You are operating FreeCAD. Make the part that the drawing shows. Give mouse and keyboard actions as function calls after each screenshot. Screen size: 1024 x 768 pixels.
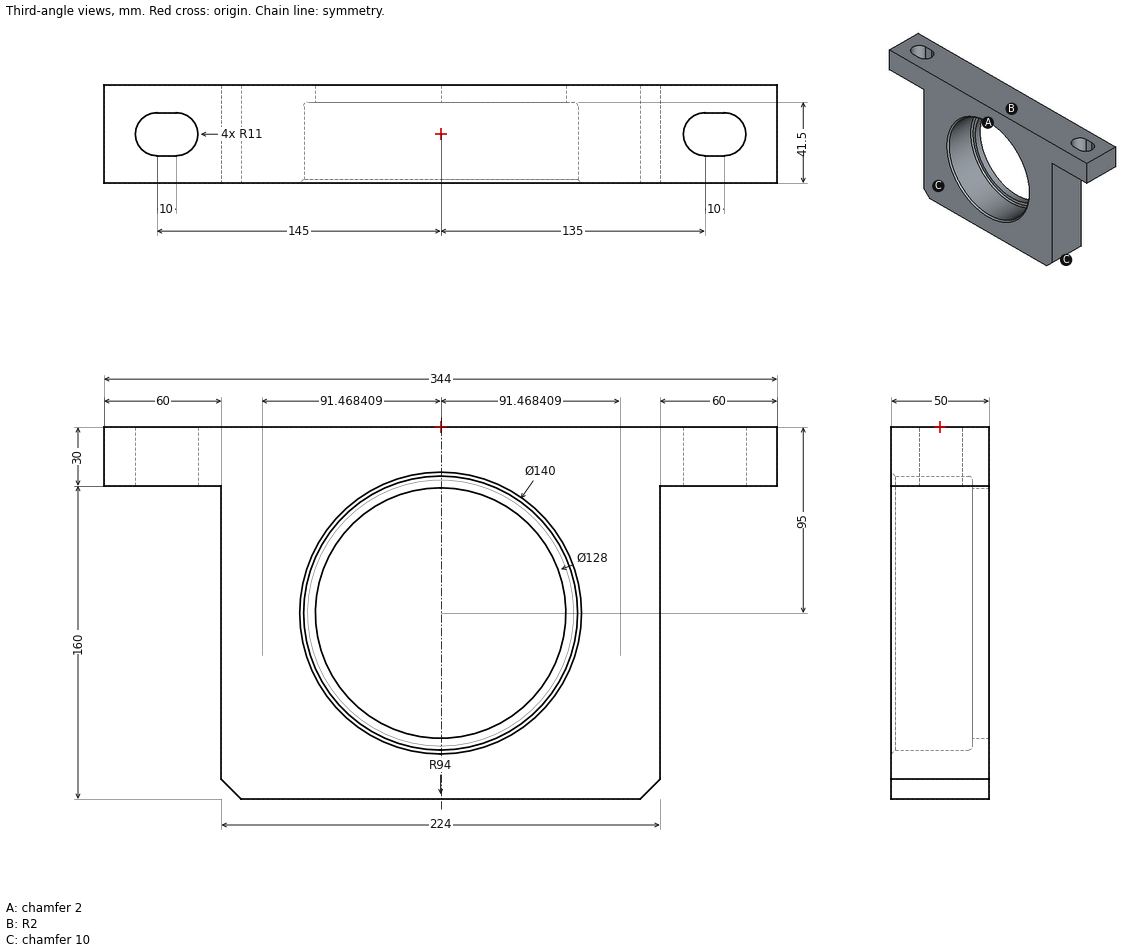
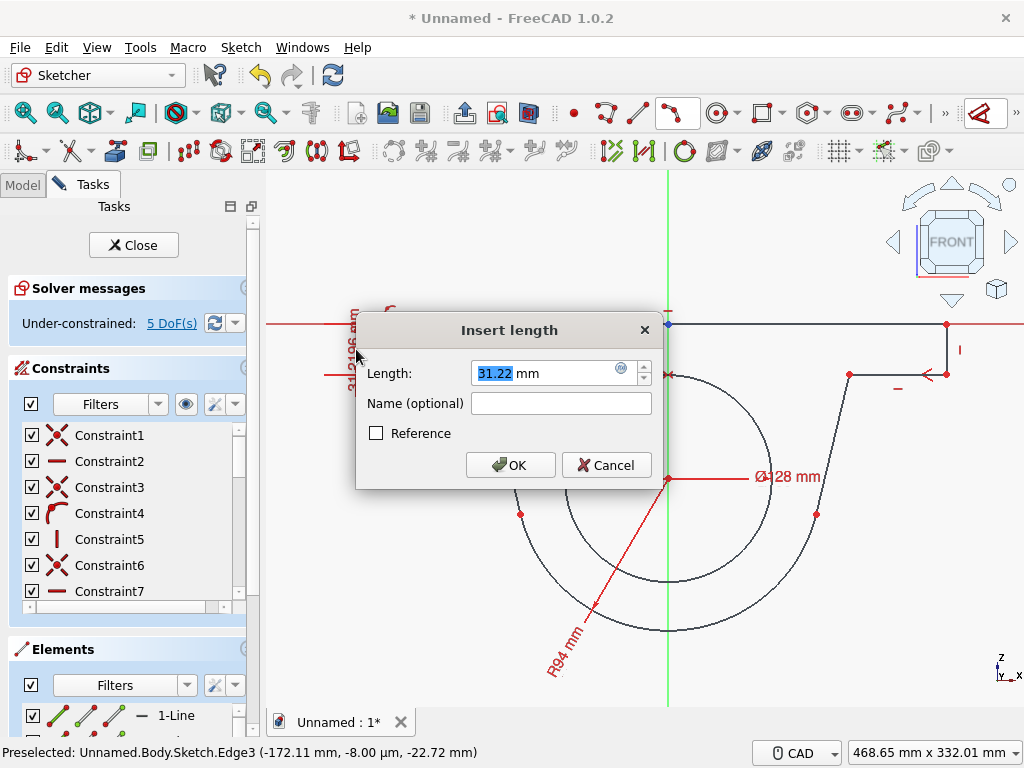
text(30)
key(Return)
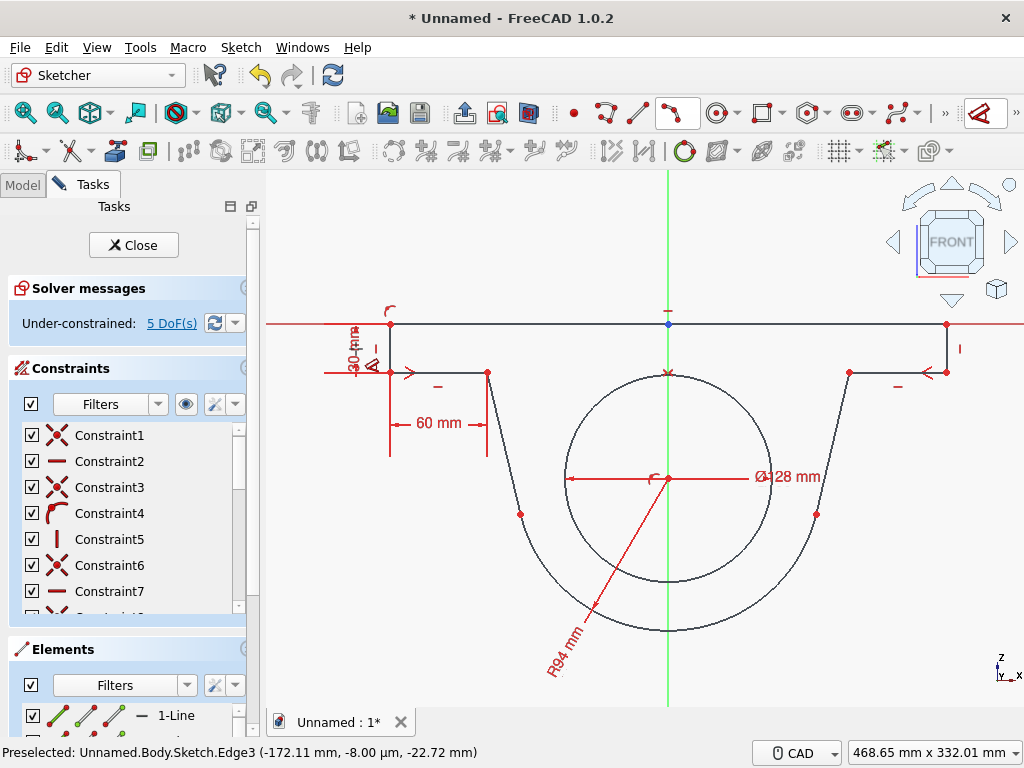
scroll(390, 360, down, 2)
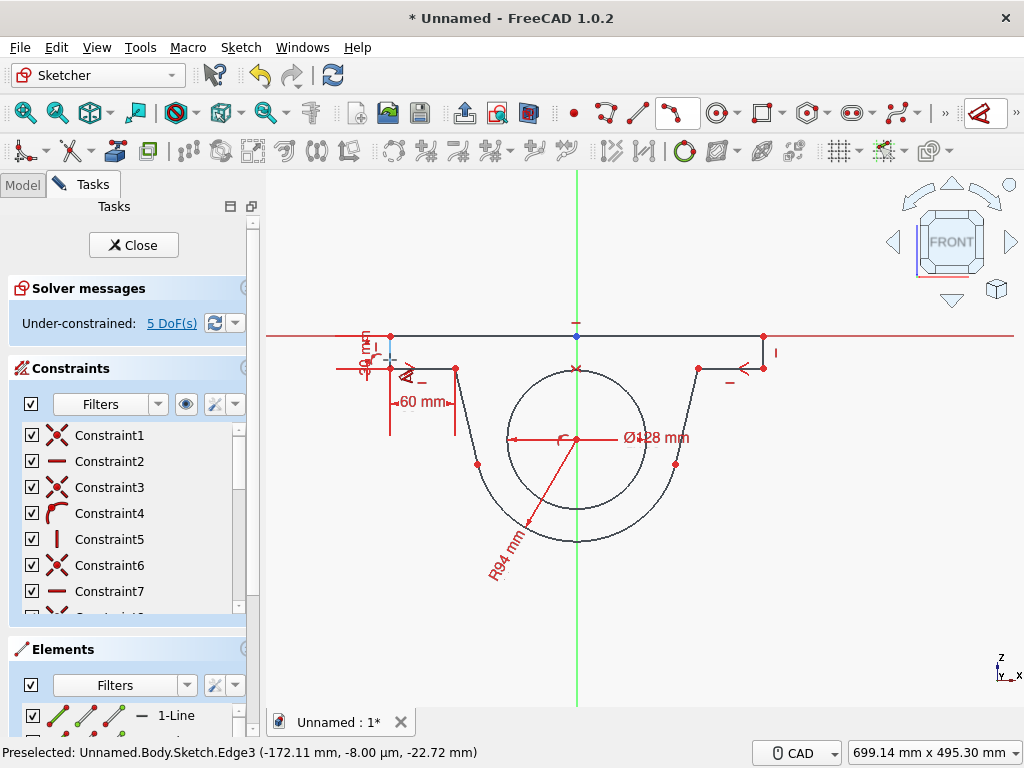
click(744, 369)
click(731, 403)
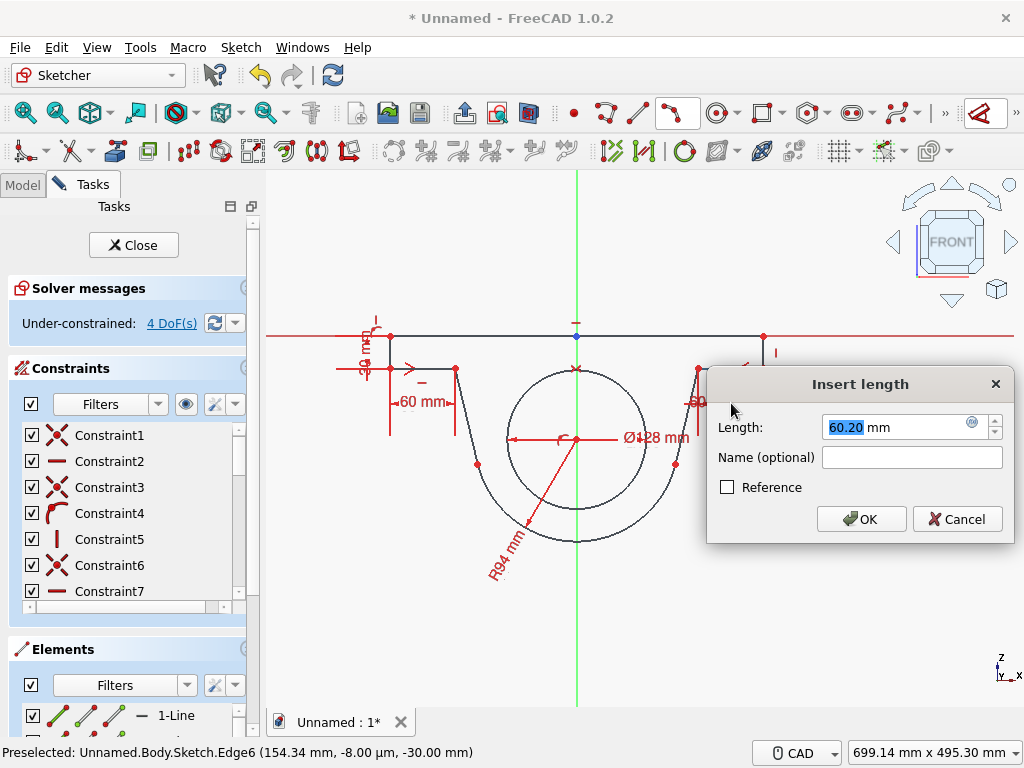
text(60)
key(Return)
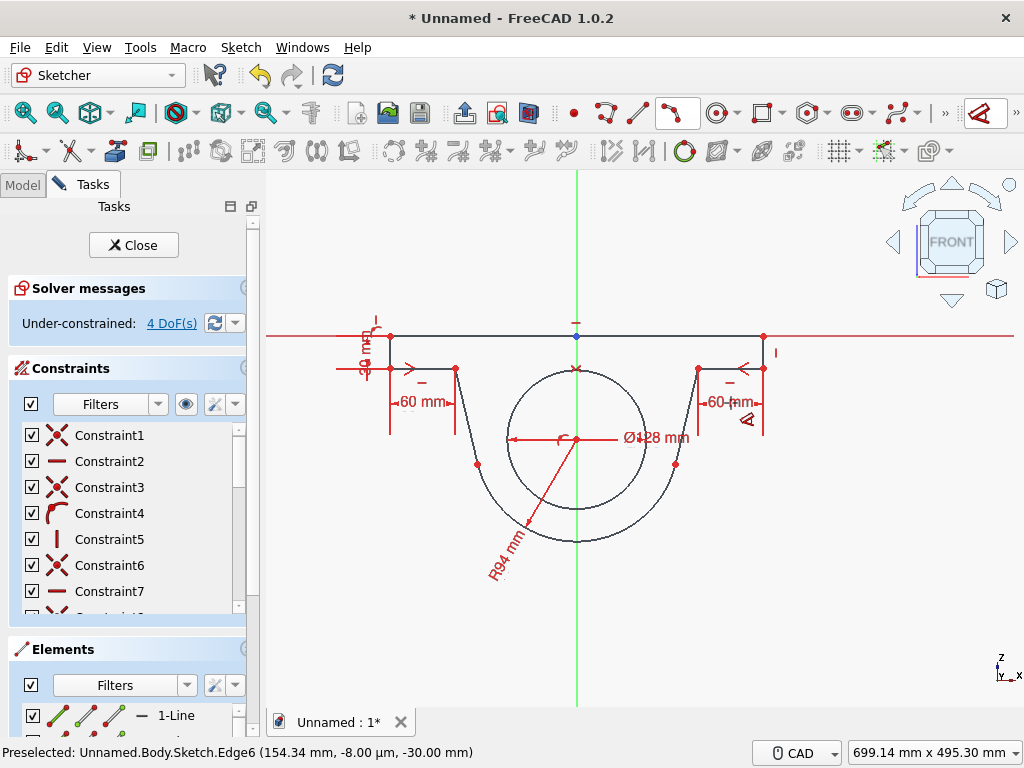
click(577, 440)
click(611, 364)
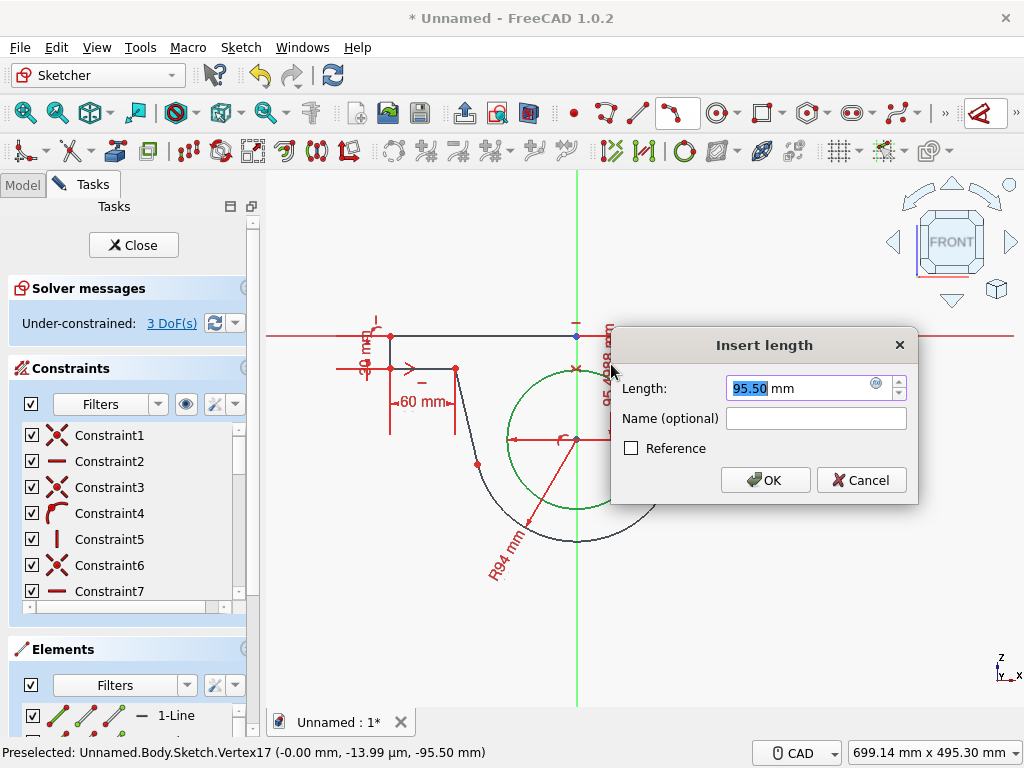
text(95)
key(Return)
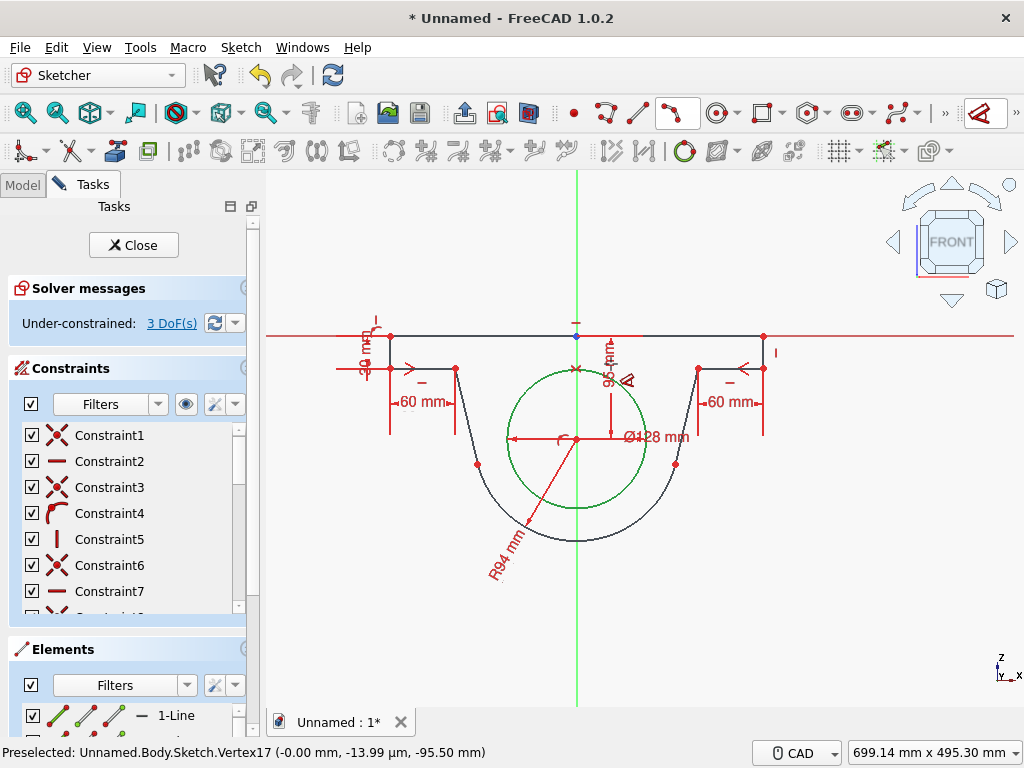
click(502, 336)
click(491, 302)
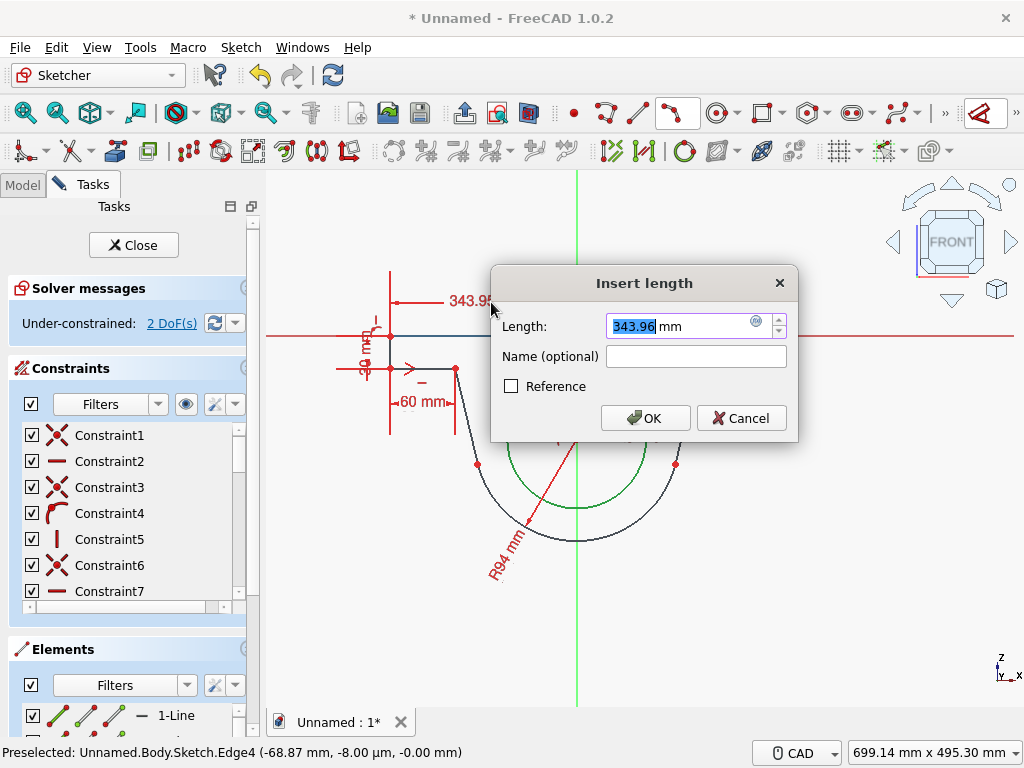
text(344)
key(Return)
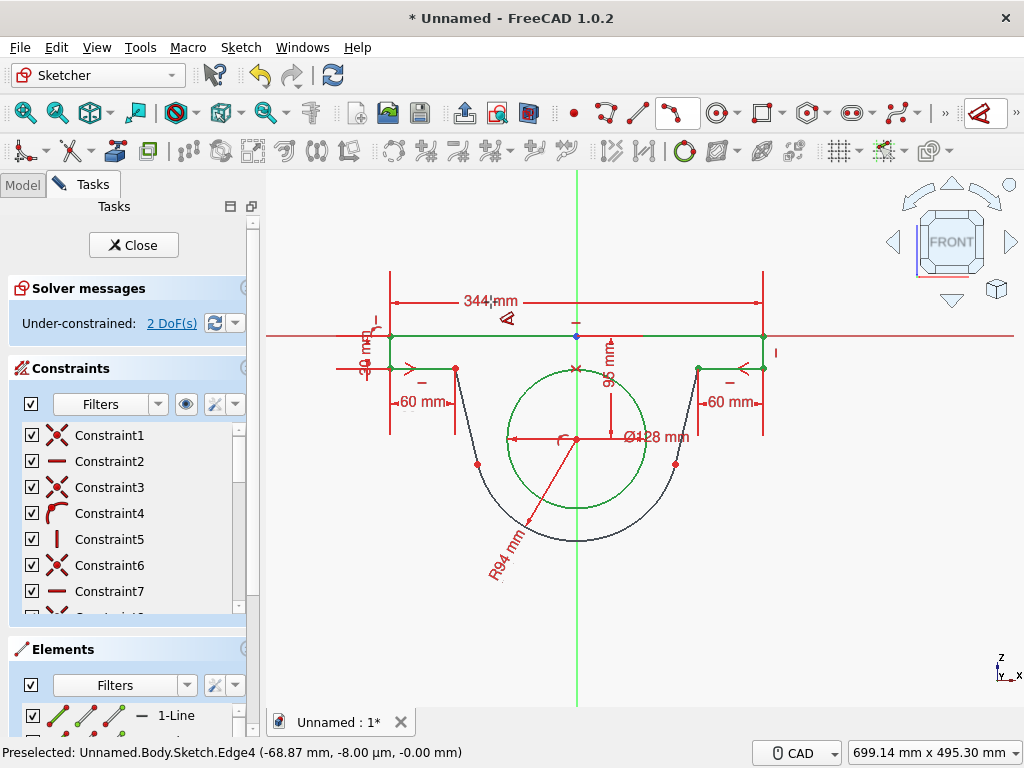
click(478, 464)
click(562, 302)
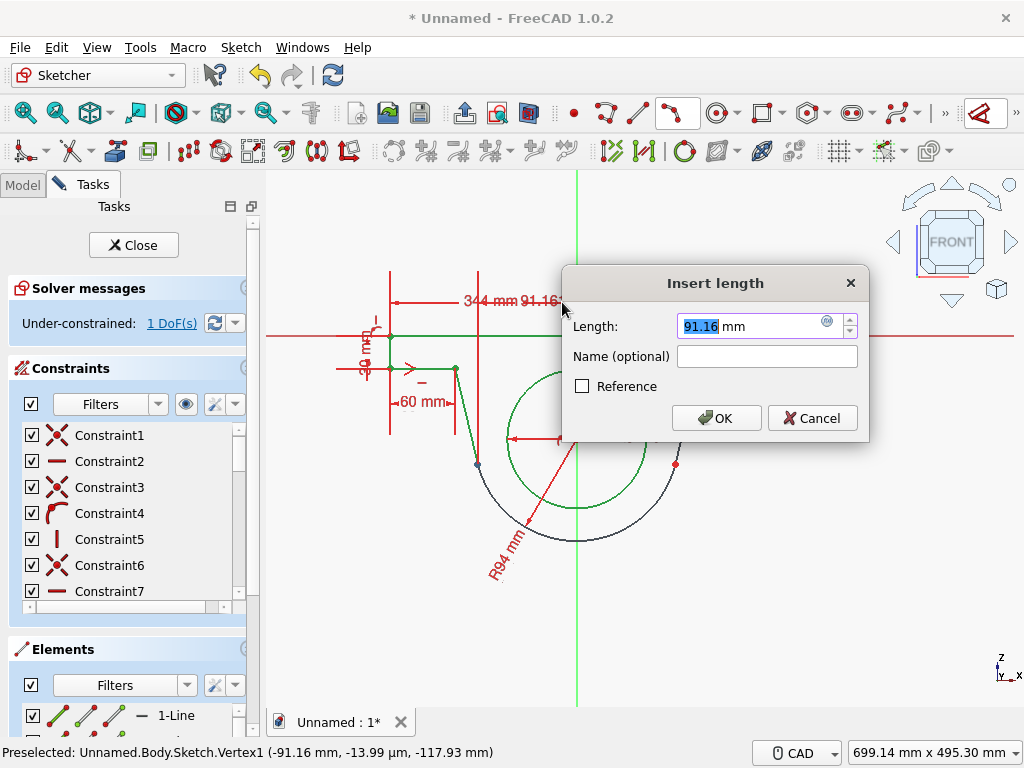
text(91.468409)
key(Return)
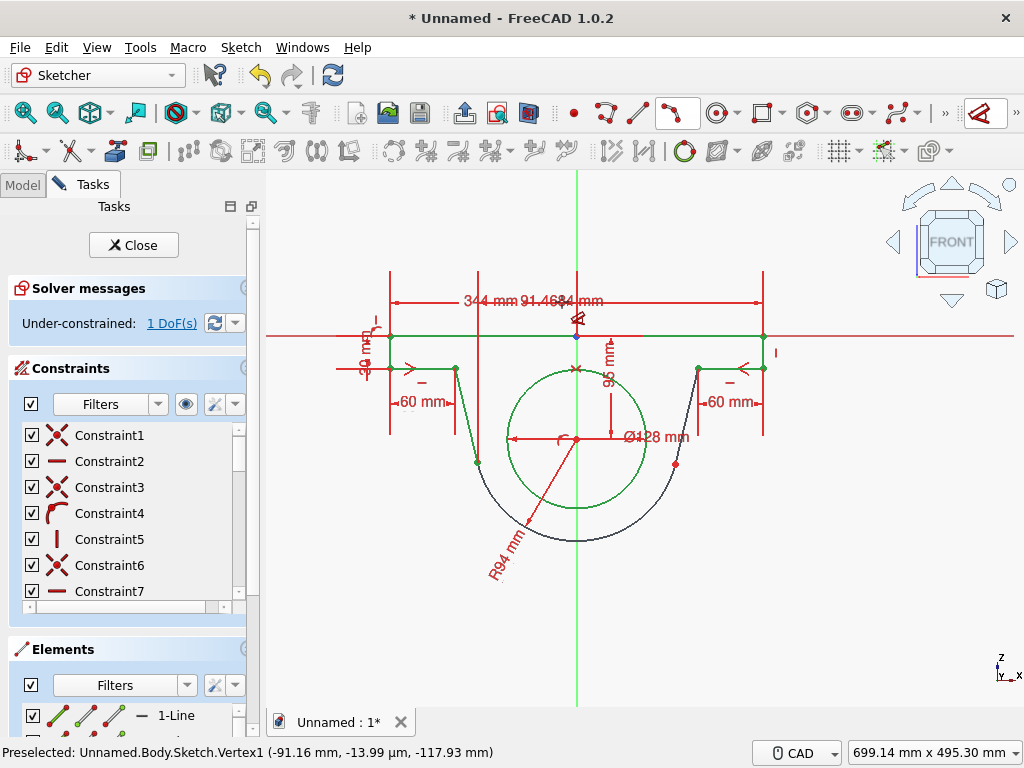
click(676, 464)
click(649, 302)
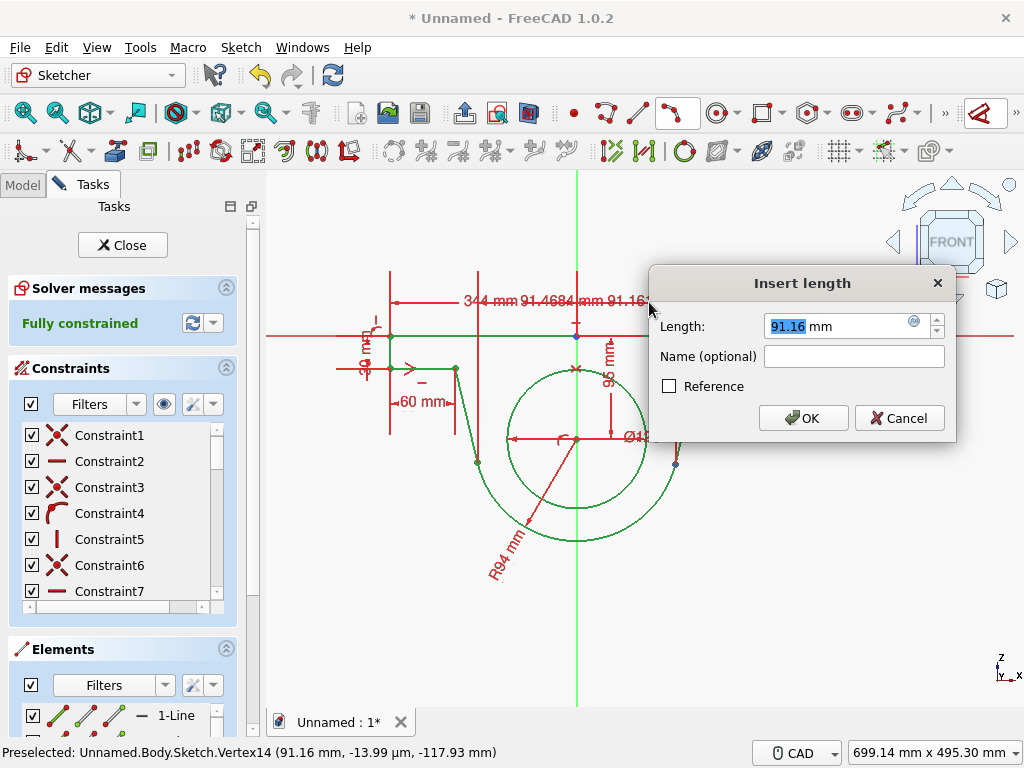
text(91.468409)
key(Return)
key(Escape)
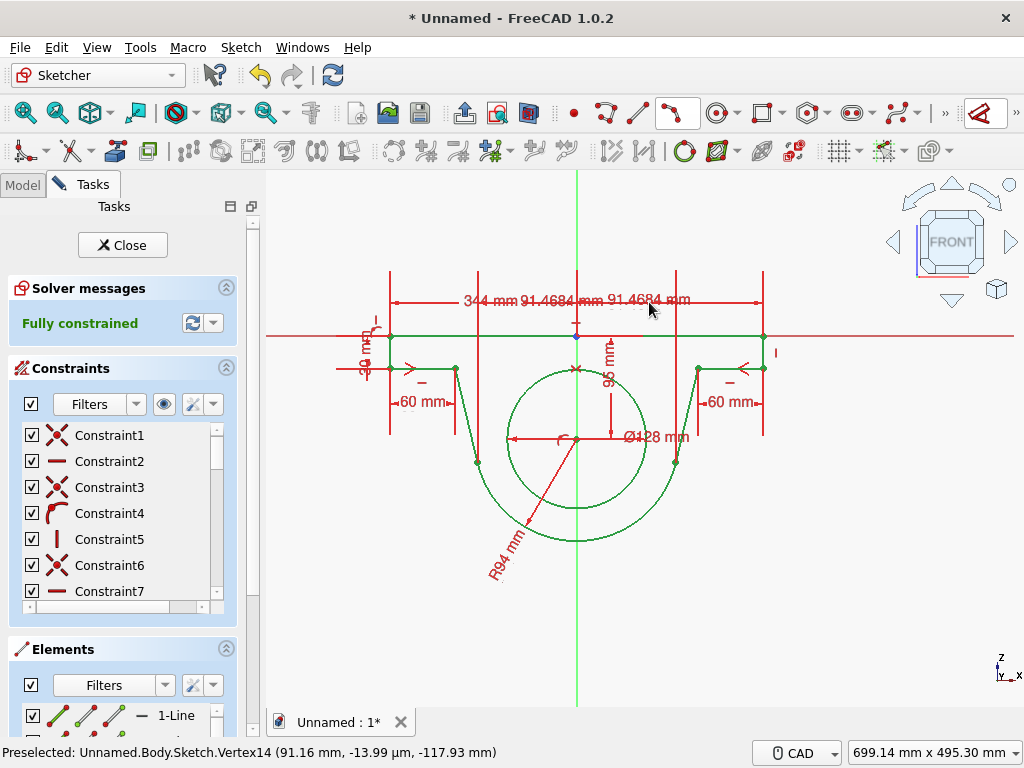
click(123, 245)